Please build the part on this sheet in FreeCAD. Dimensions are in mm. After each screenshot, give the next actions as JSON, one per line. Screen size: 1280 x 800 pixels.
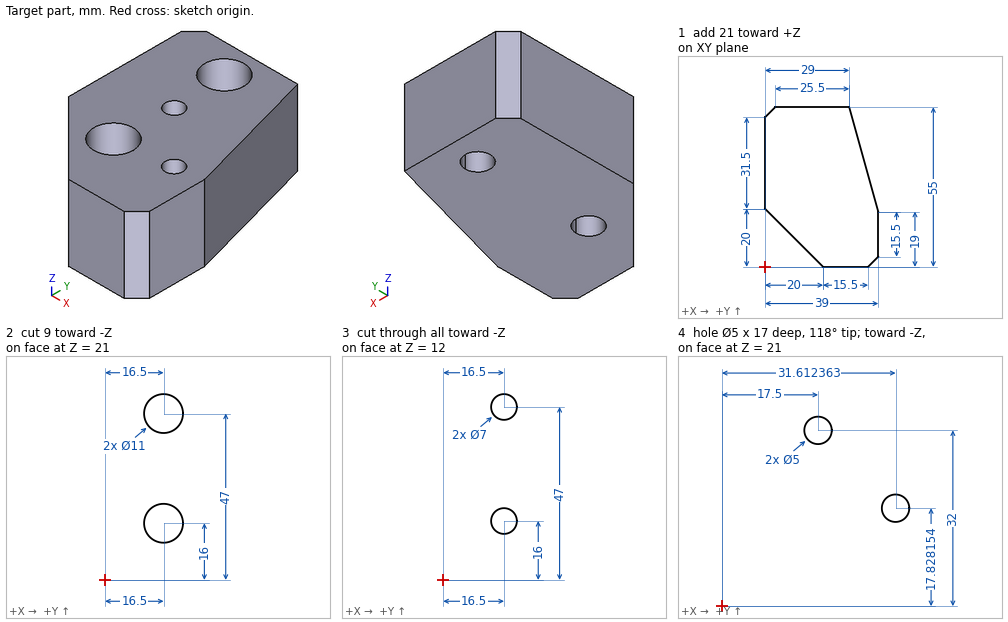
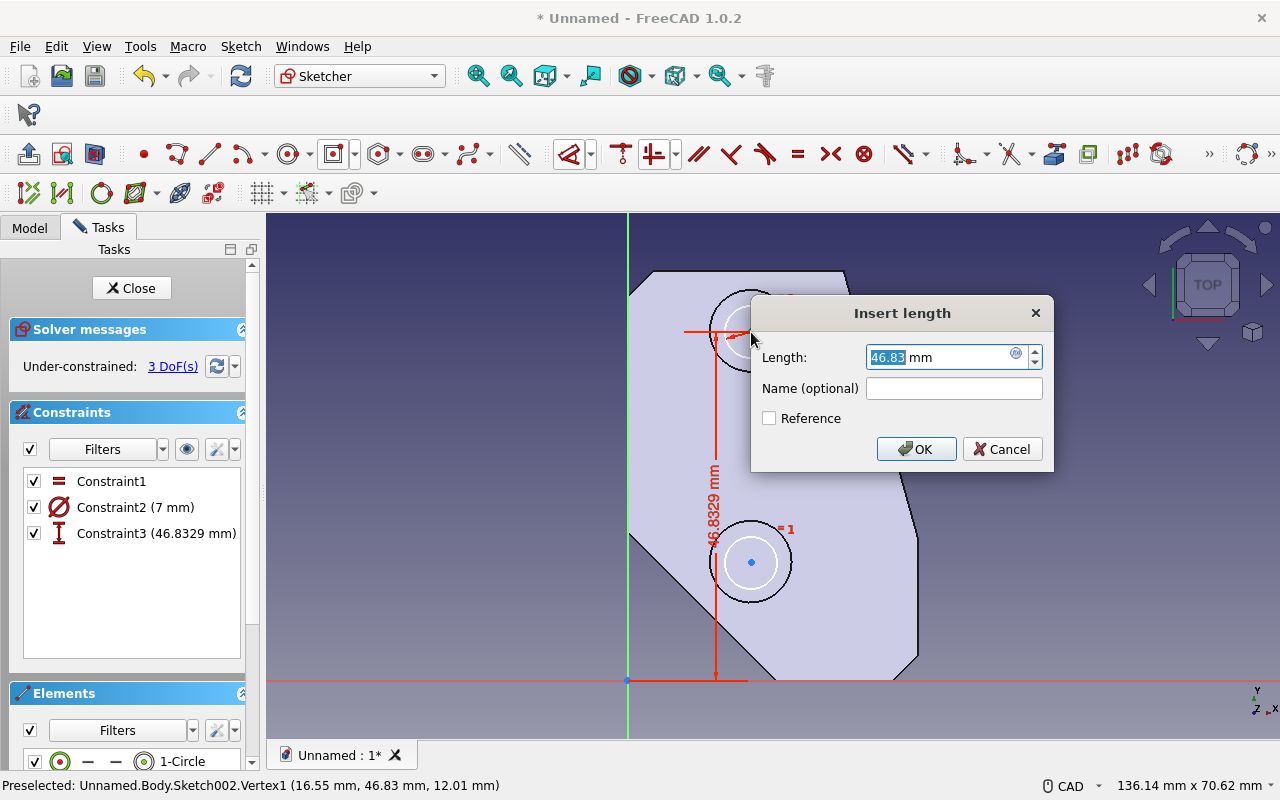
{"action": "type", "text": "47"}
{"action": "key", "text": "Return"}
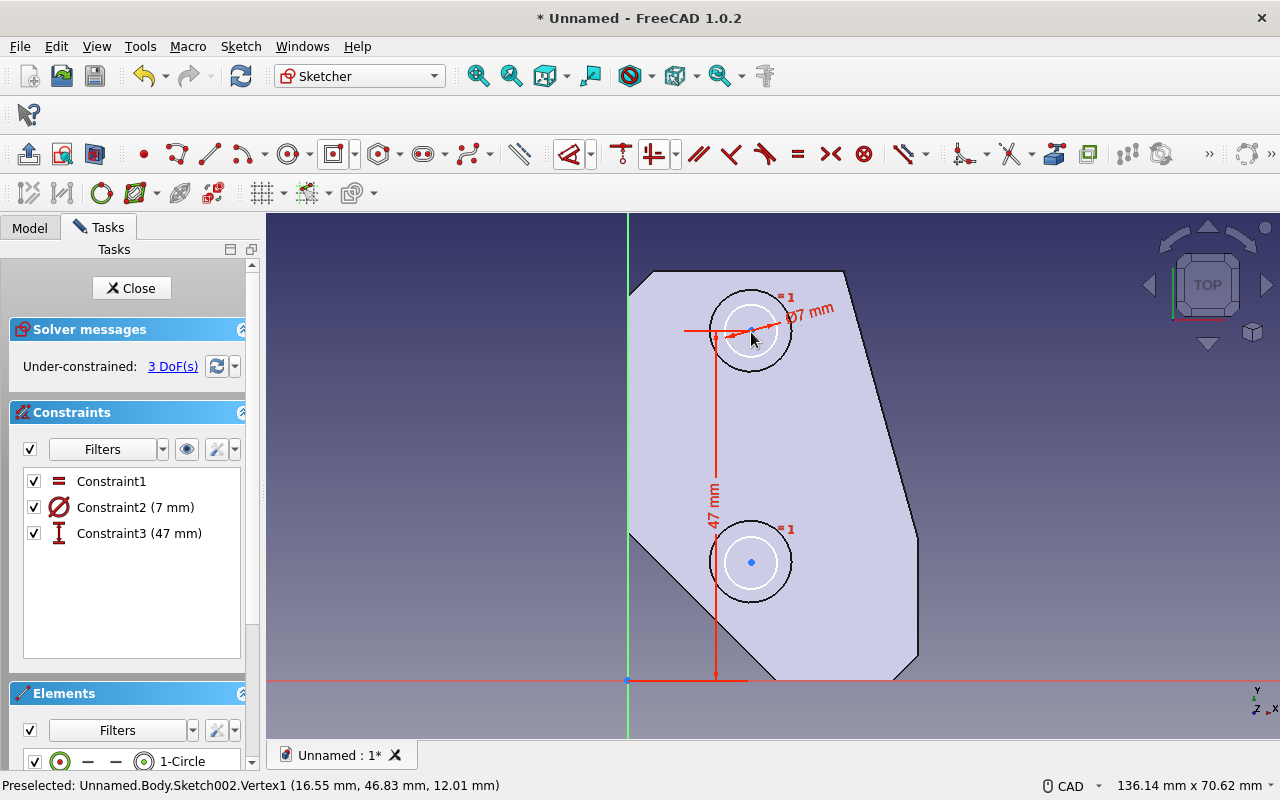
{"action": "left_click", "coordinate": [751, 563]}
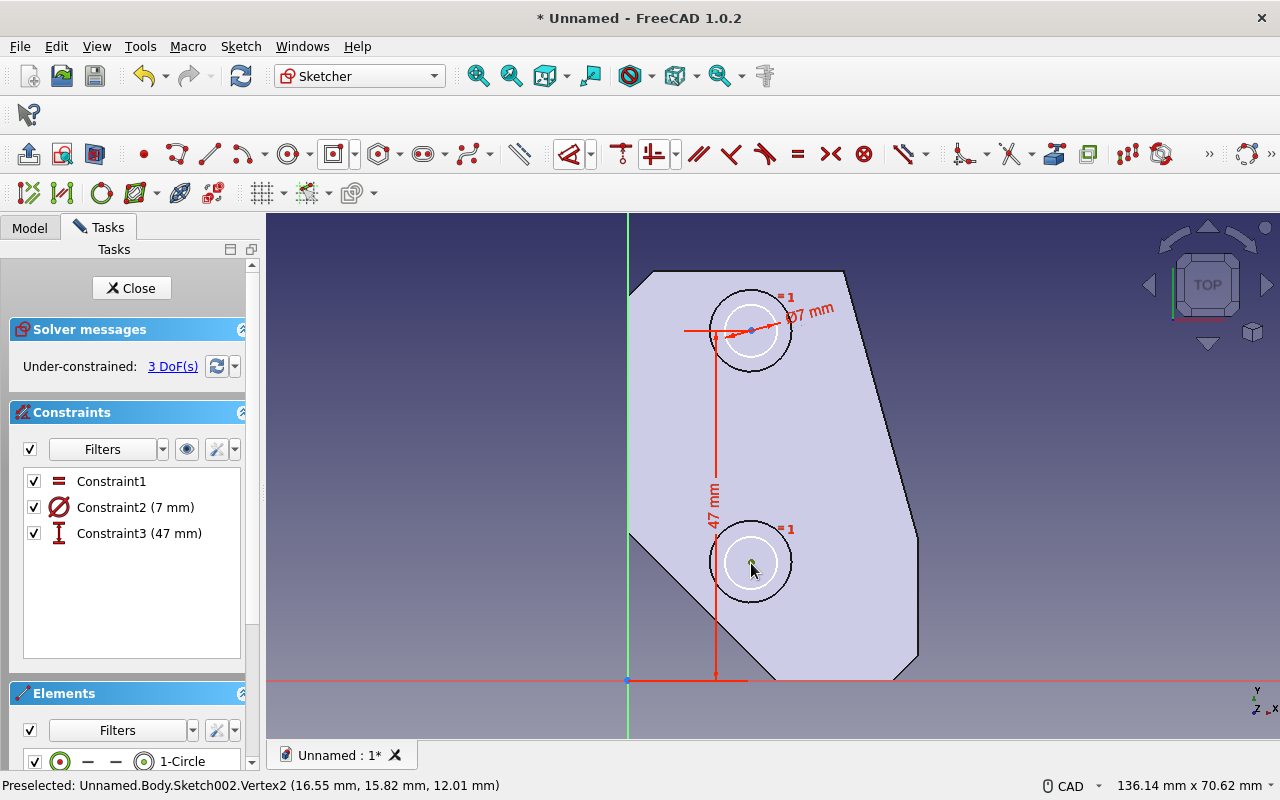
{"action": "left_click", "coordinate": [590, 154]}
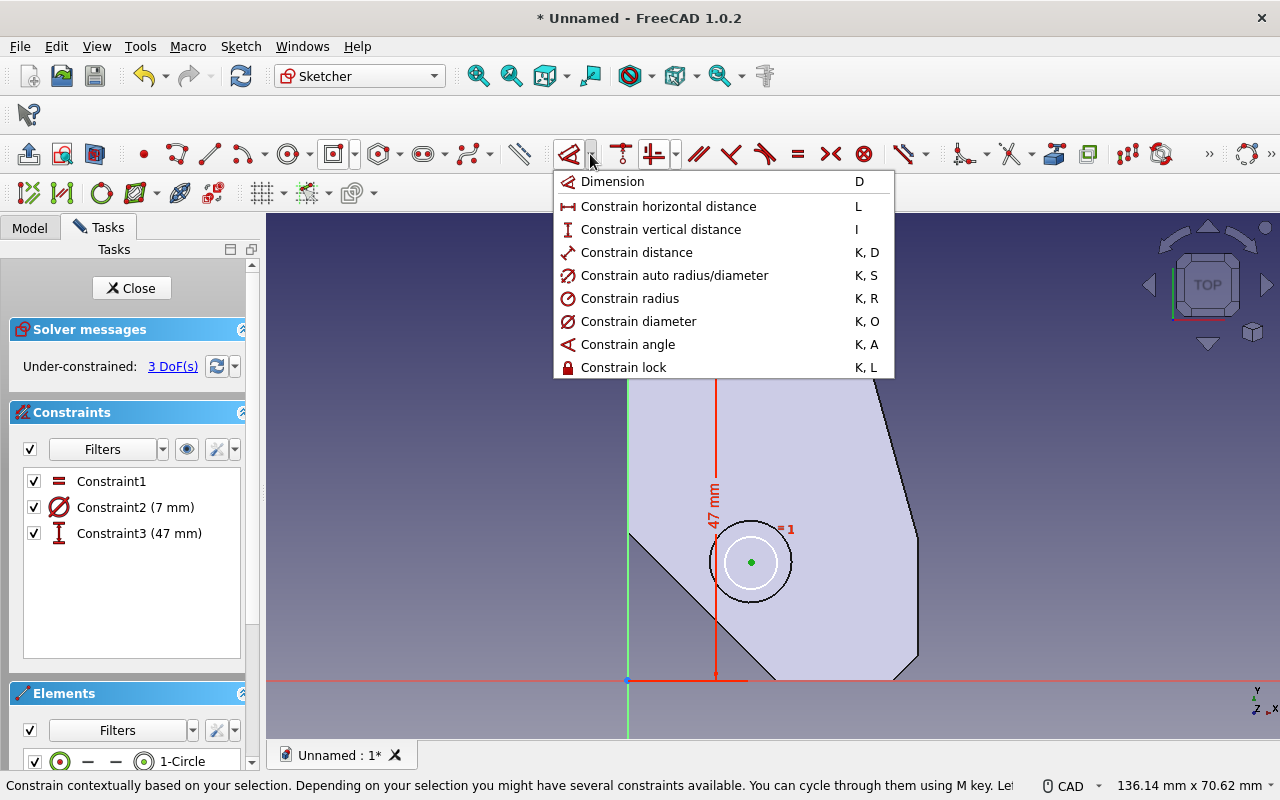
{"action": "left_click", "coordinate": [724, 230]}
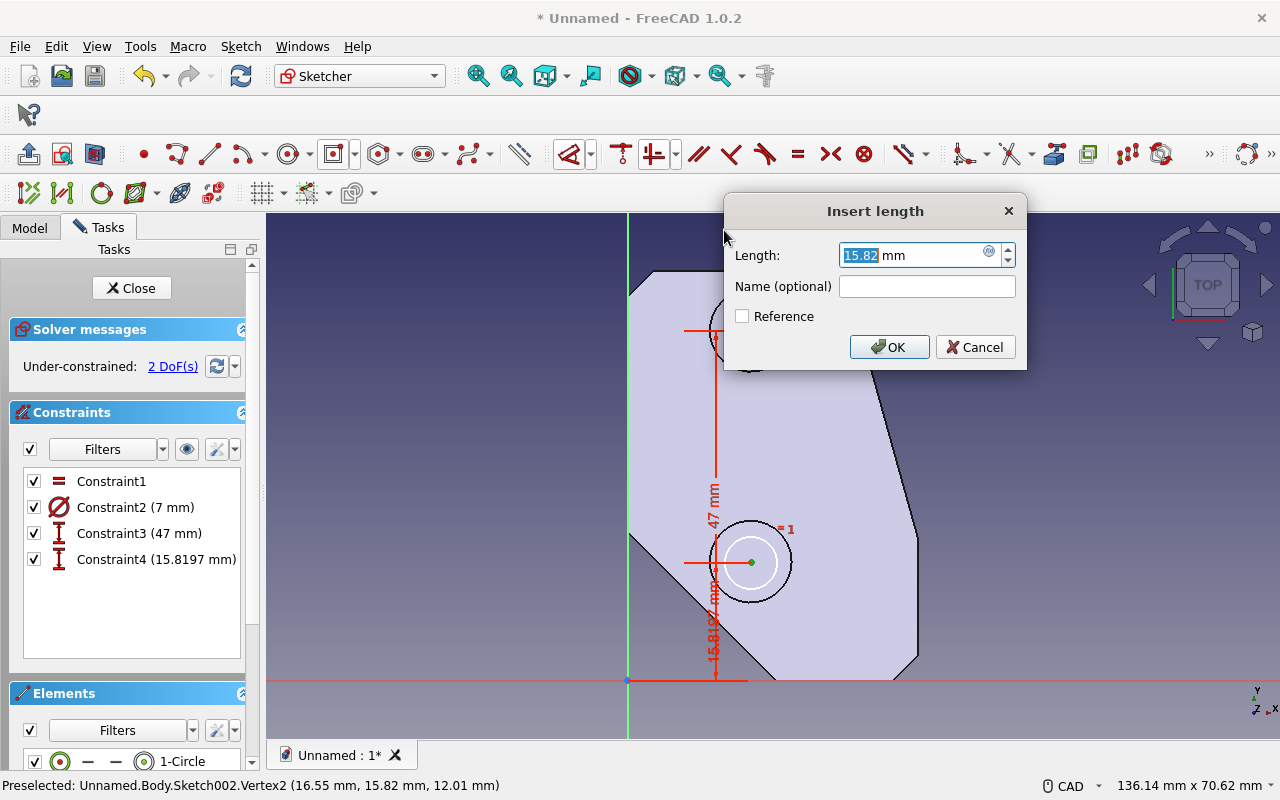
{"action": "type", "text": "16"}
{"action": "key", "text": "Return"}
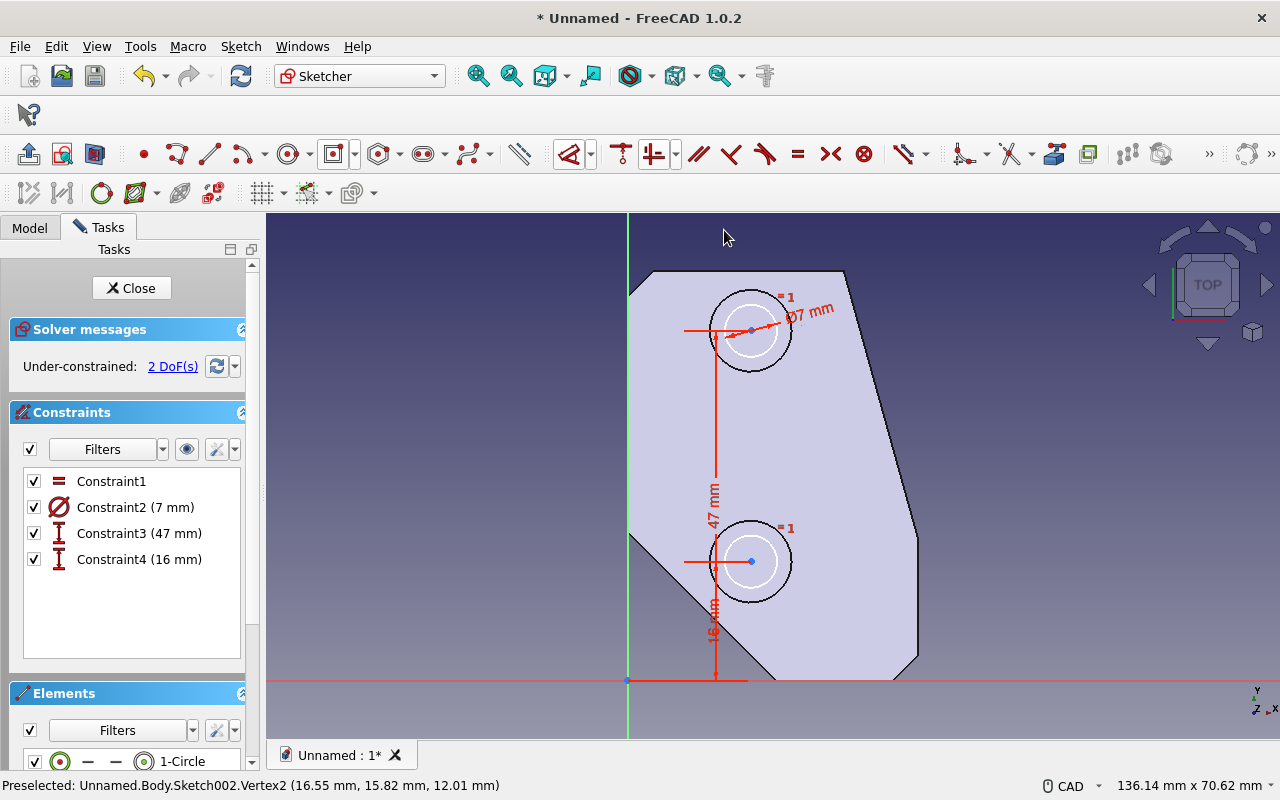
{"action": "left_click", "coordinate": [751, 331]}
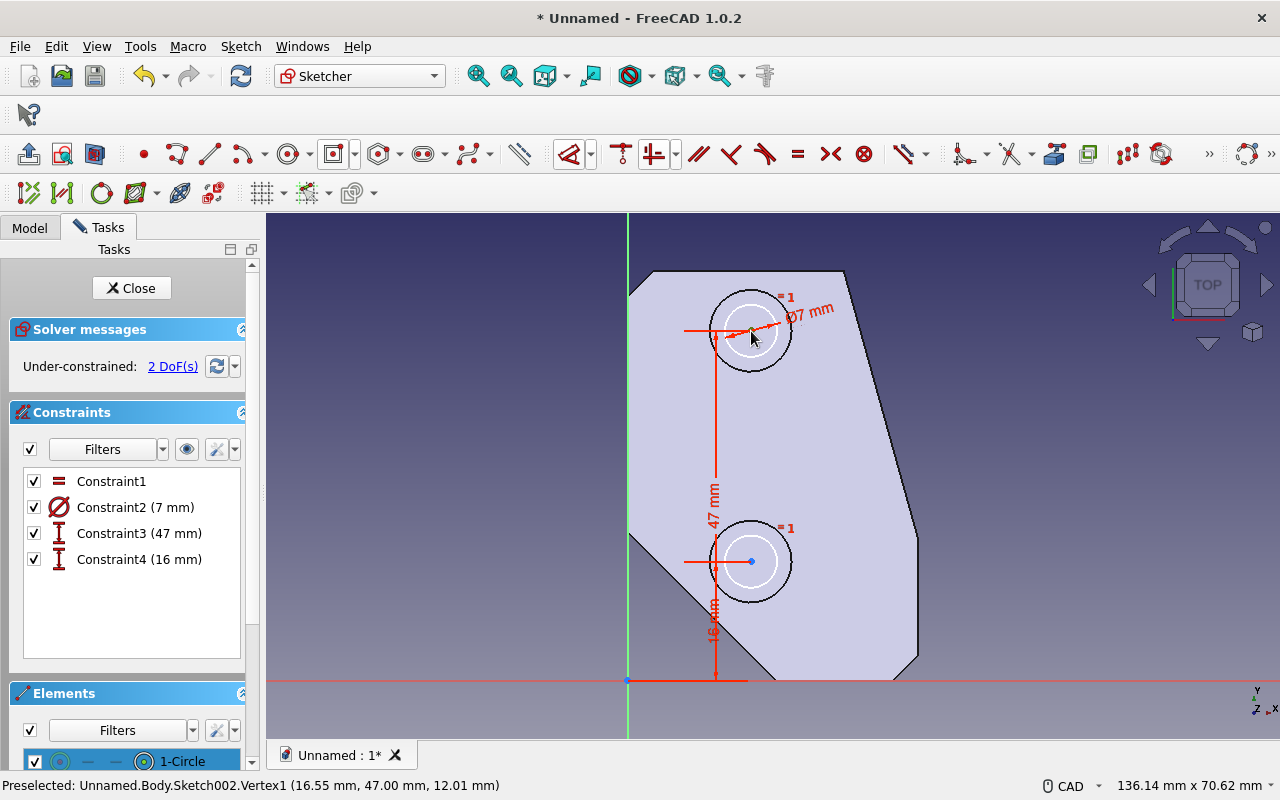
{"action": "key", "text": "l"}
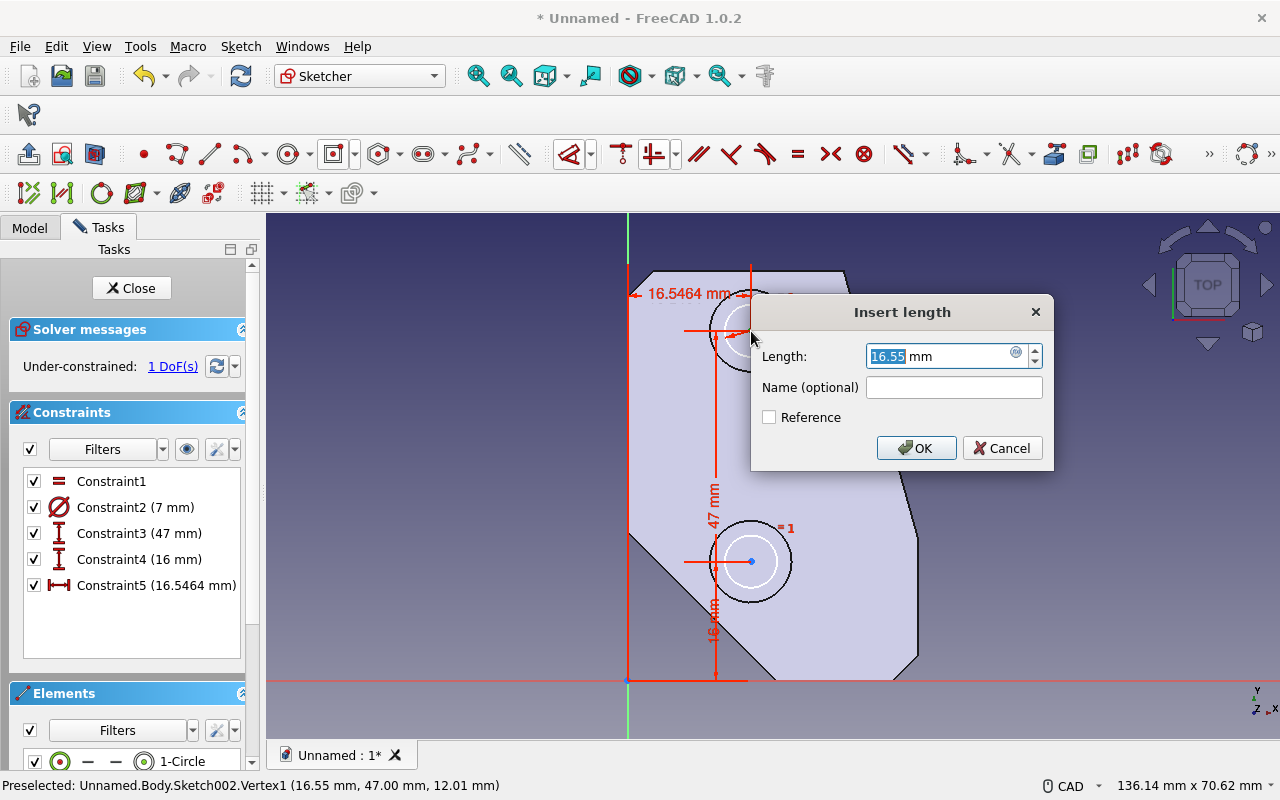
{"action": "type", "text": "16.5"}
{"action": "key", "text": "Return"}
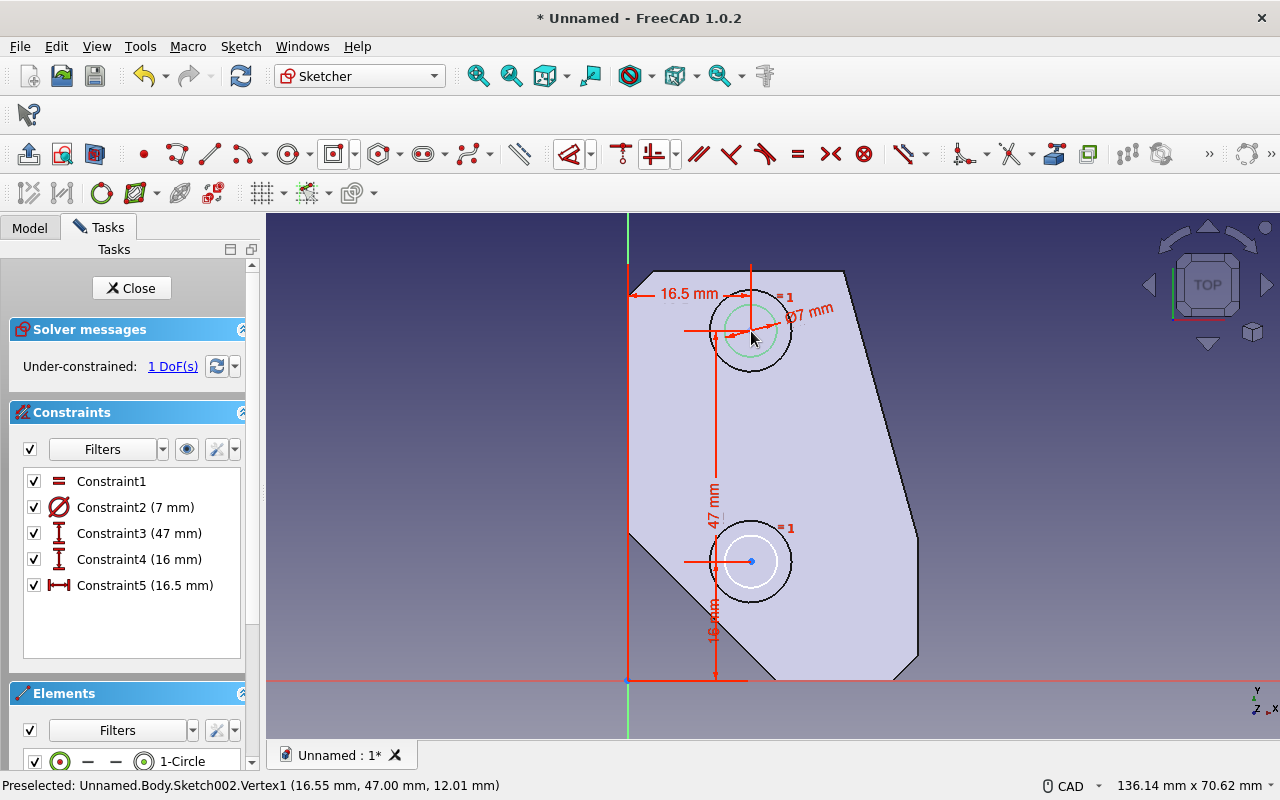
{"action": "left_click", "coordinate": [751, 562]}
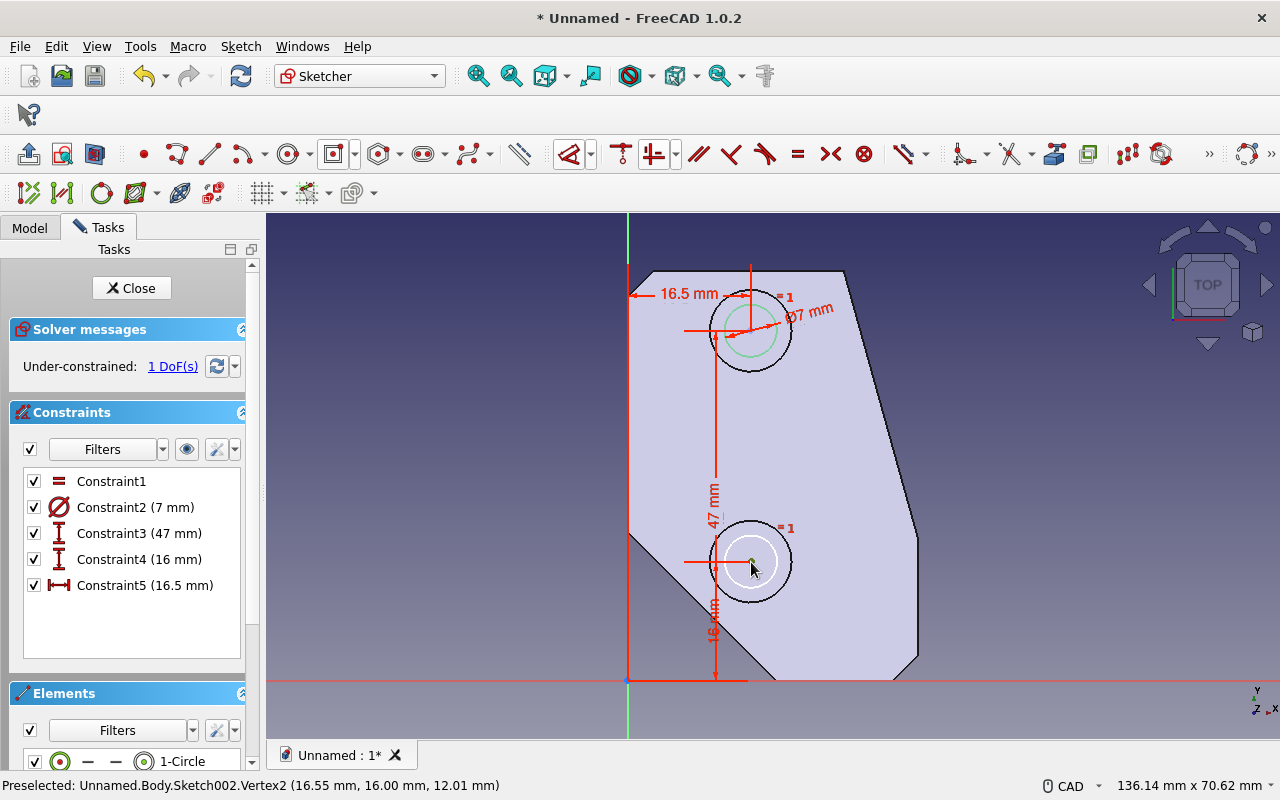
{"action": "key", "text": "l"}